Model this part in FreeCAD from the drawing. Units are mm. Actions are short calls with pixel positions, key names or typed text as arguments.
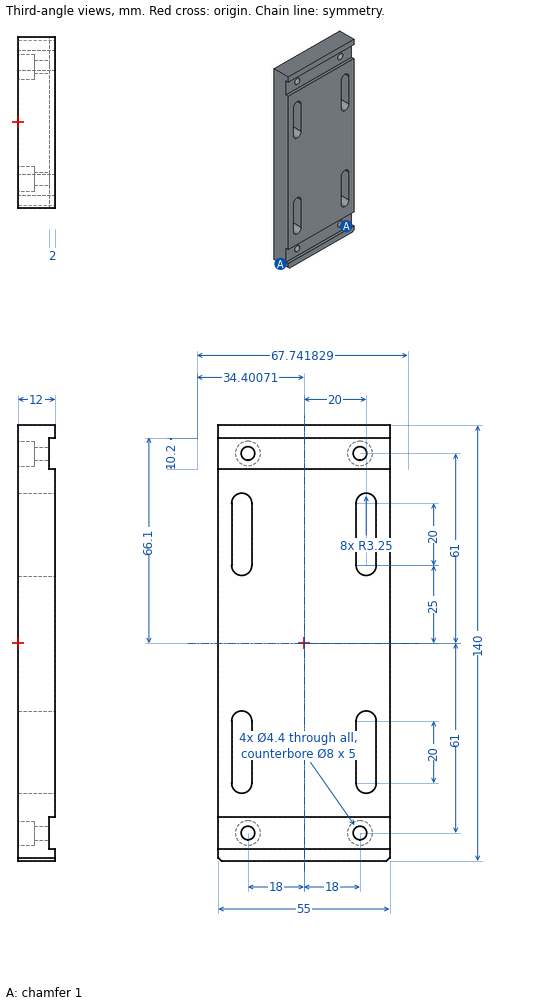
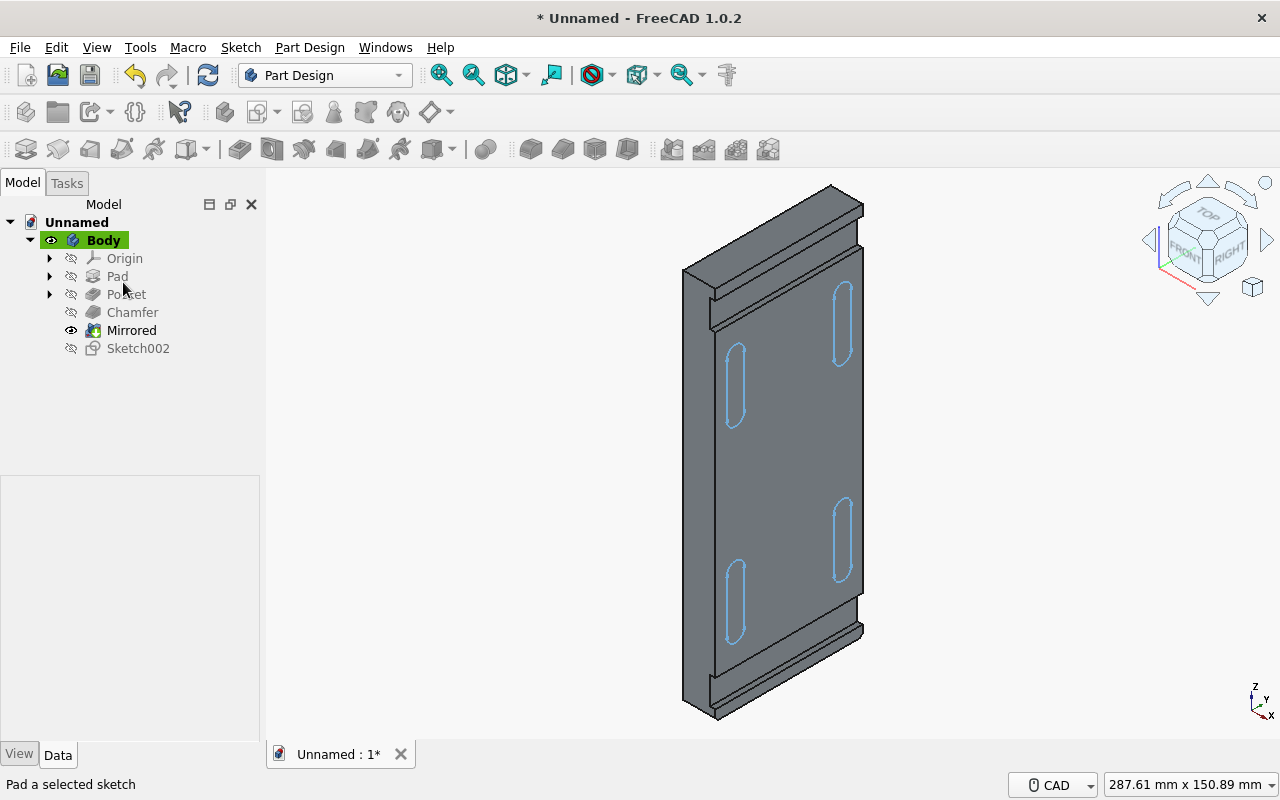
click(240, 150)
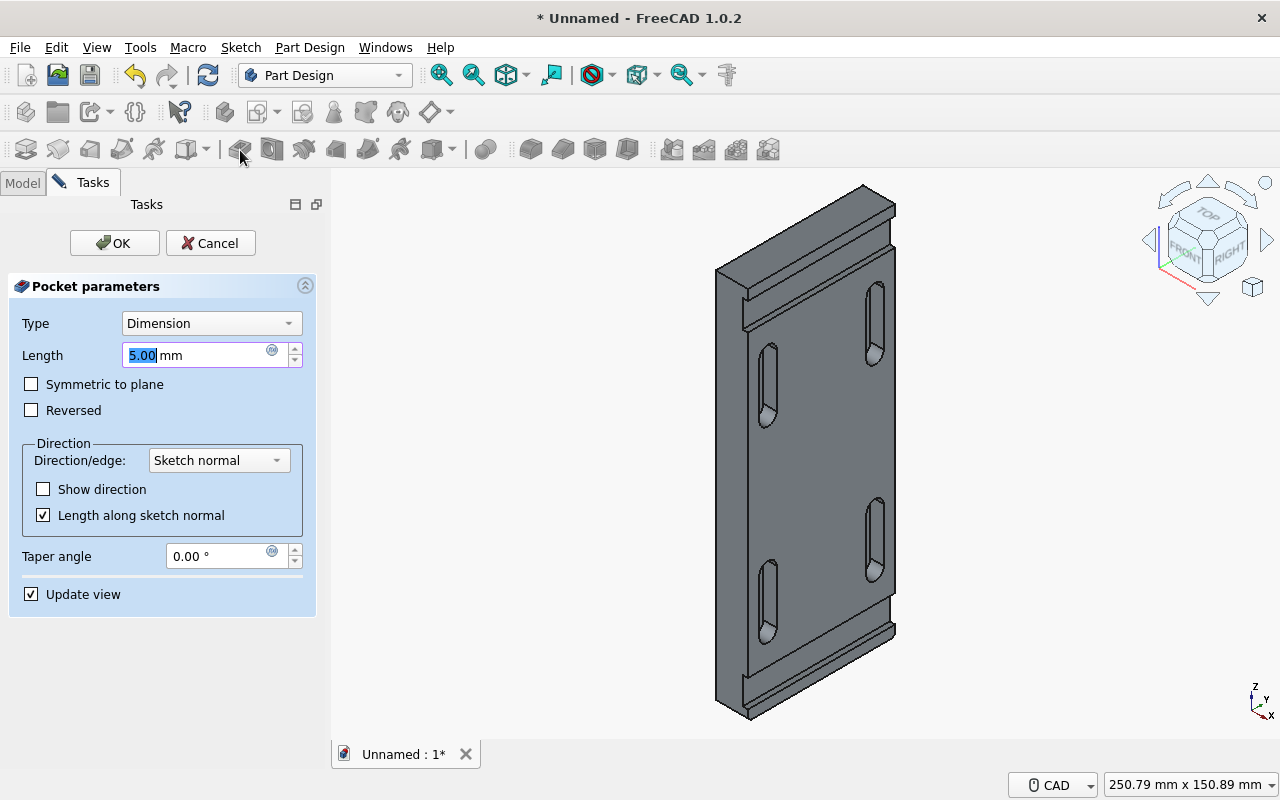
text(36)
key(Tab)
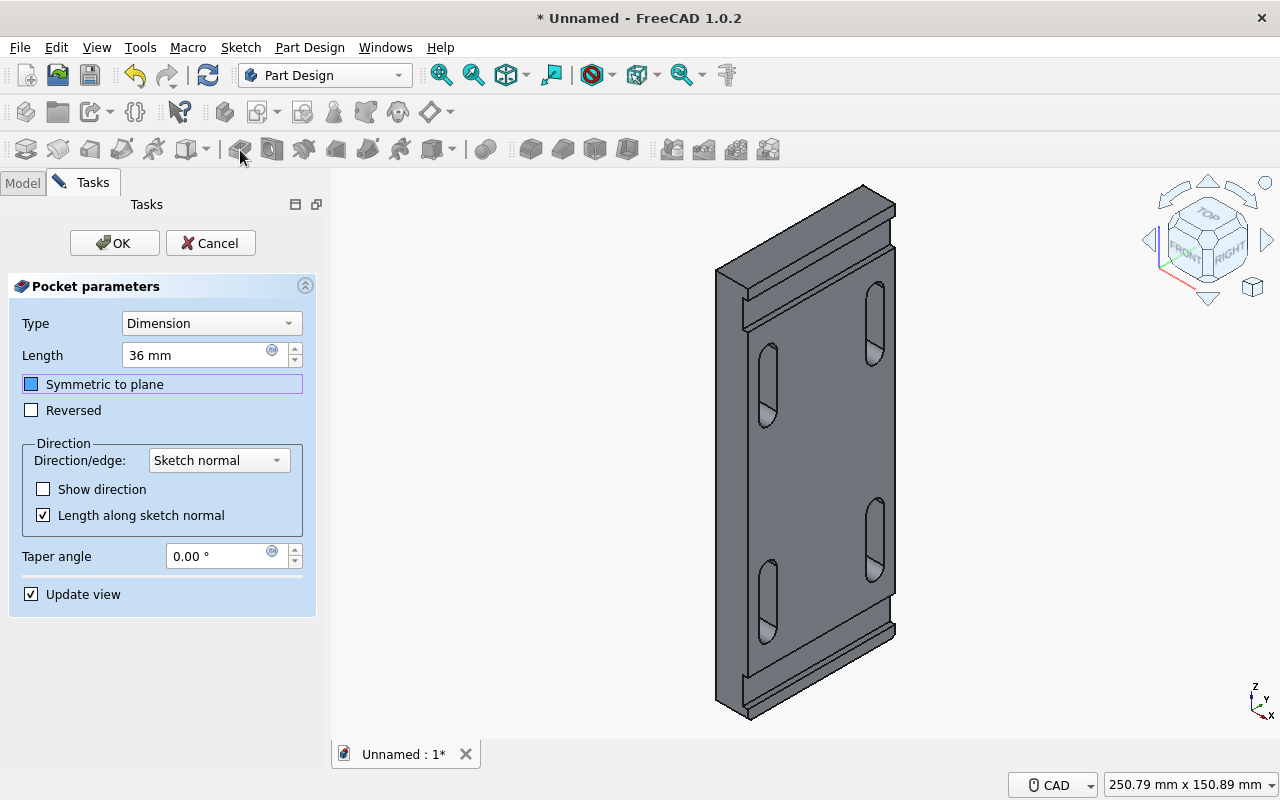
click(115, 243)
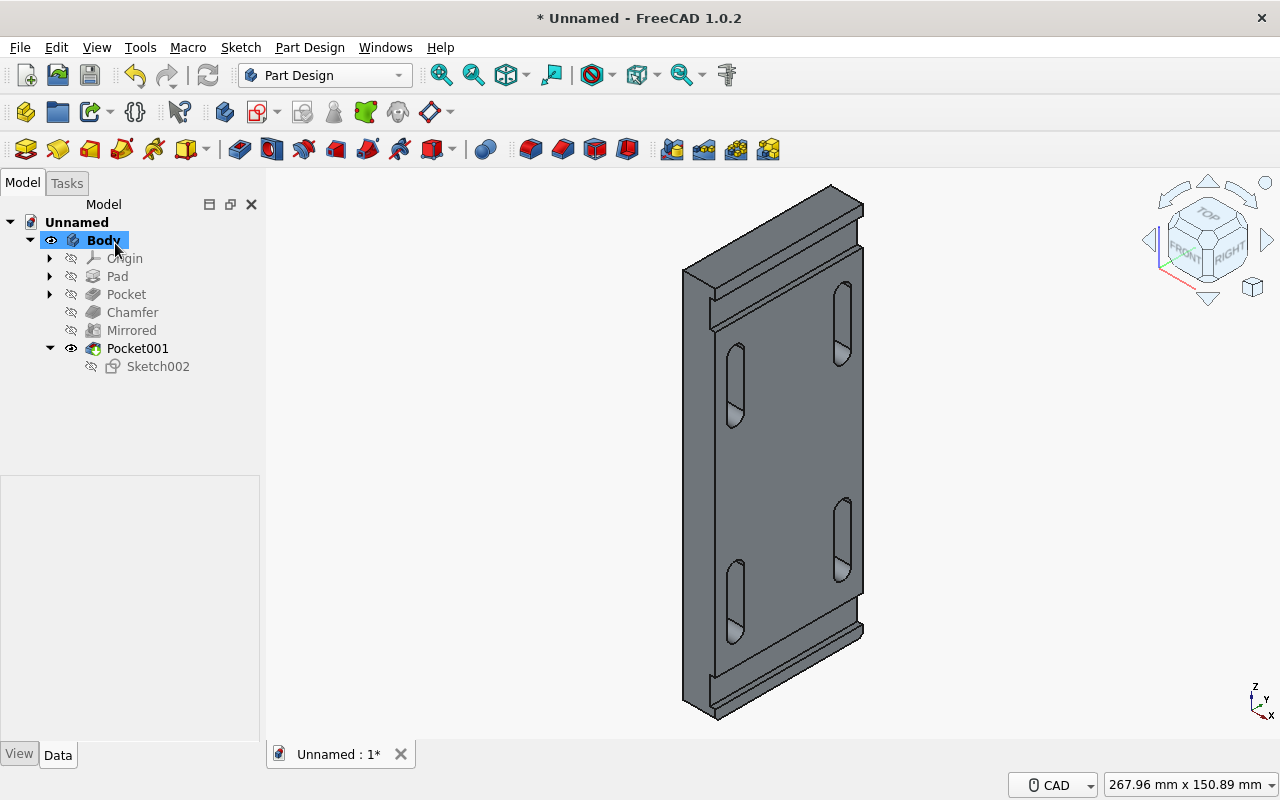
click(258, 112)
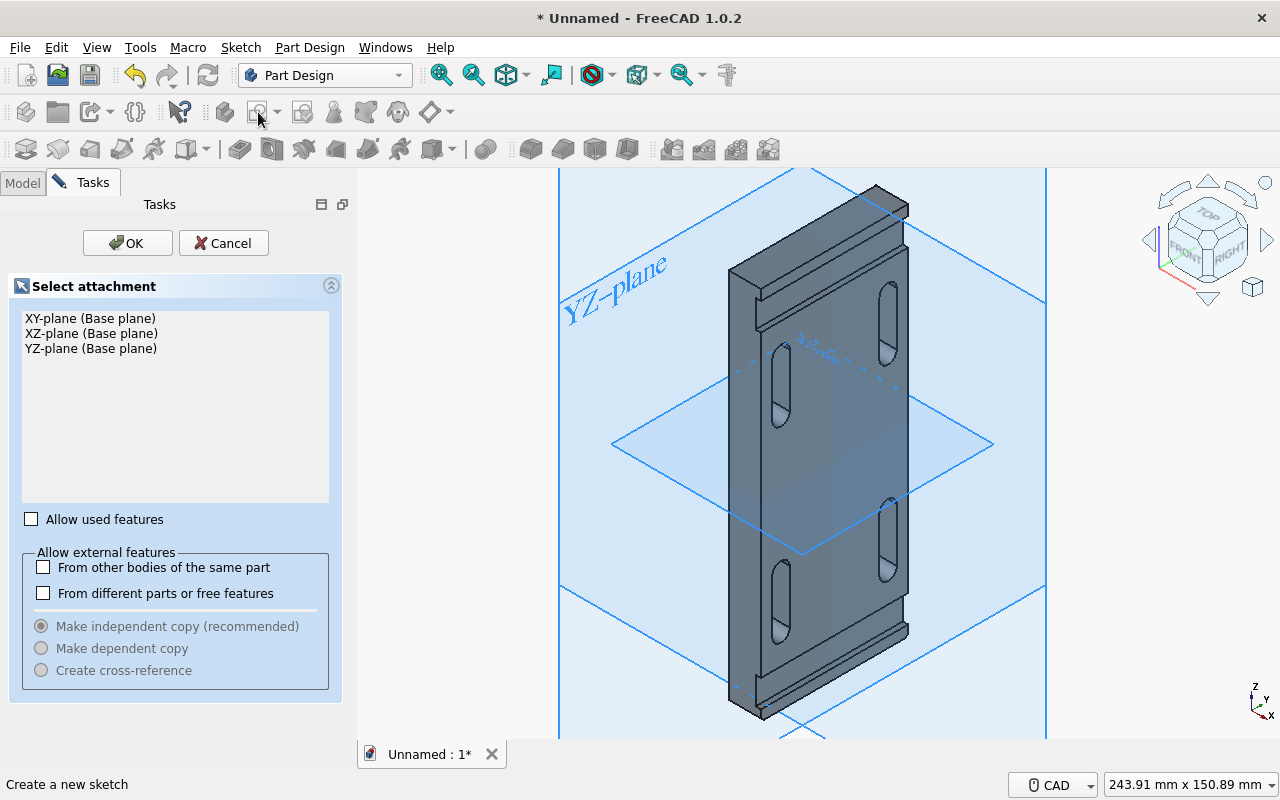
click(82, 348)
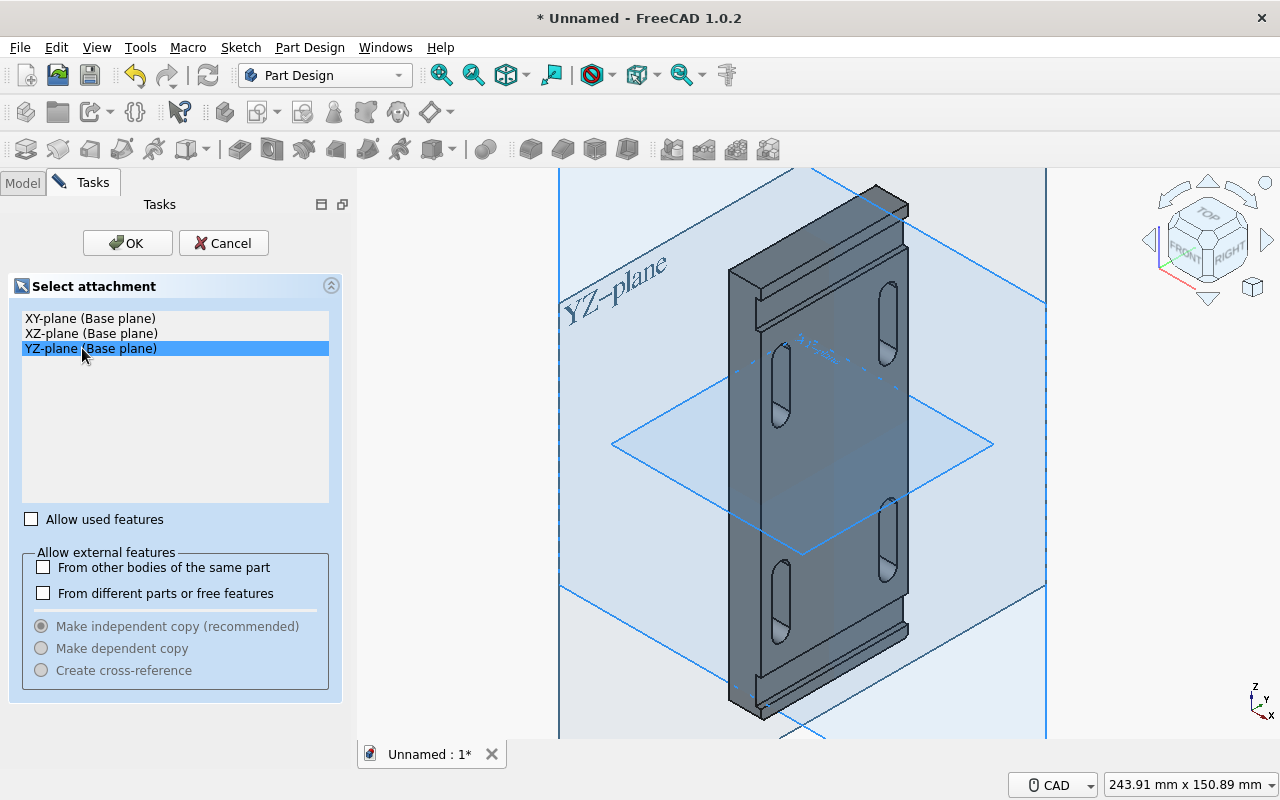
click(128, 243)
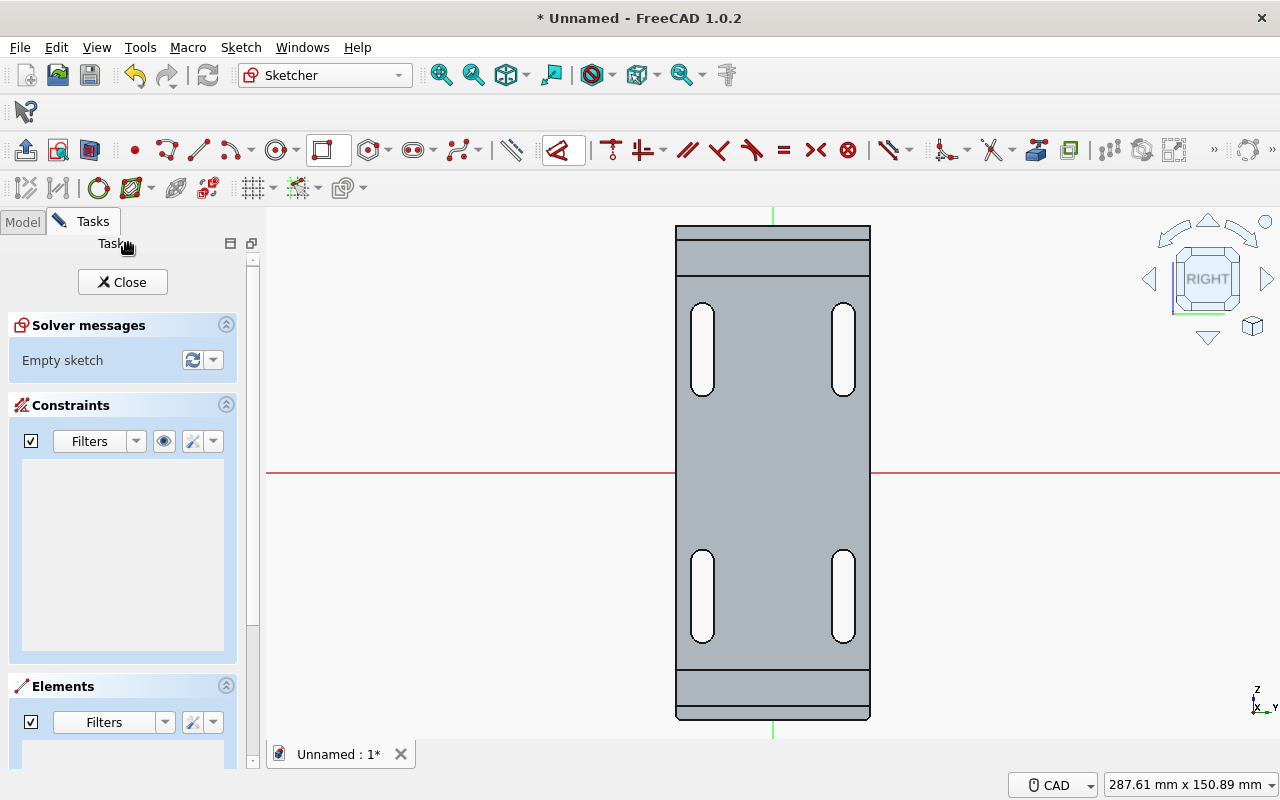
click(90, 150)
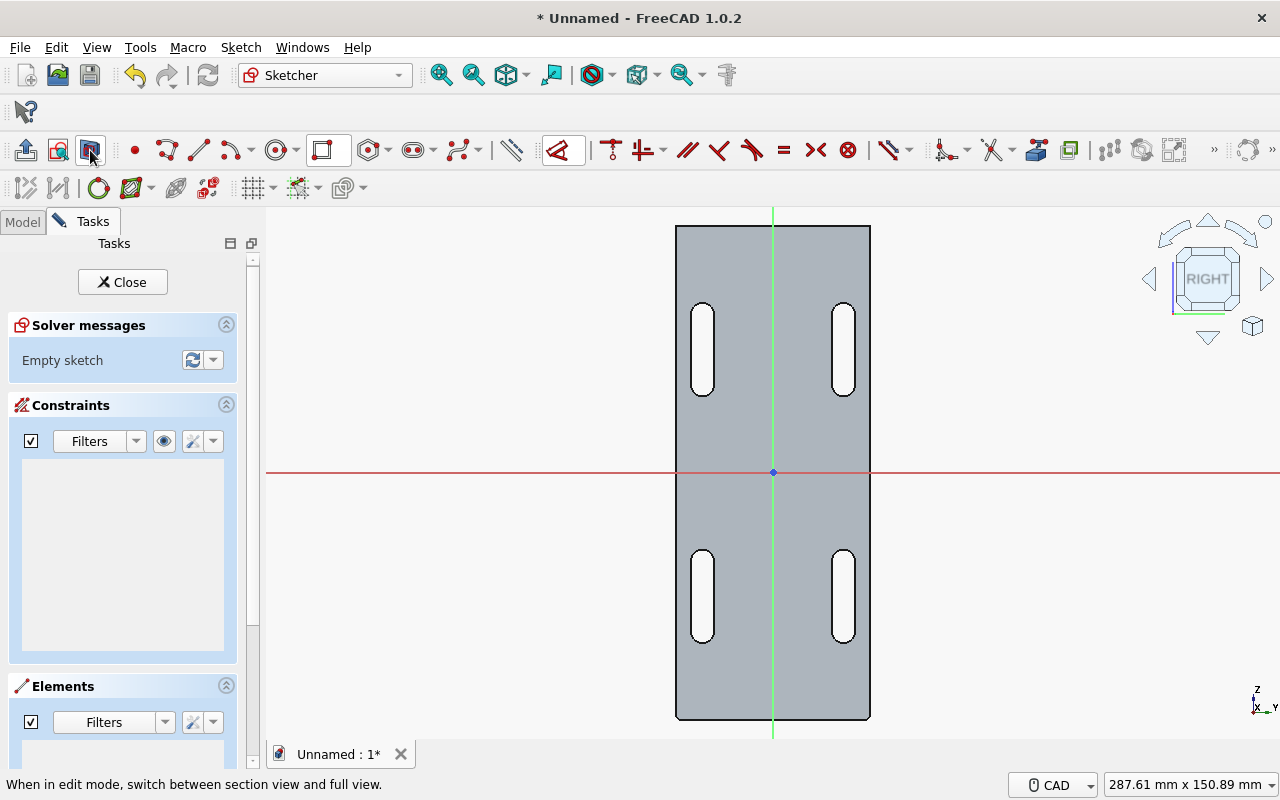
scroll(395, 473, down, 1)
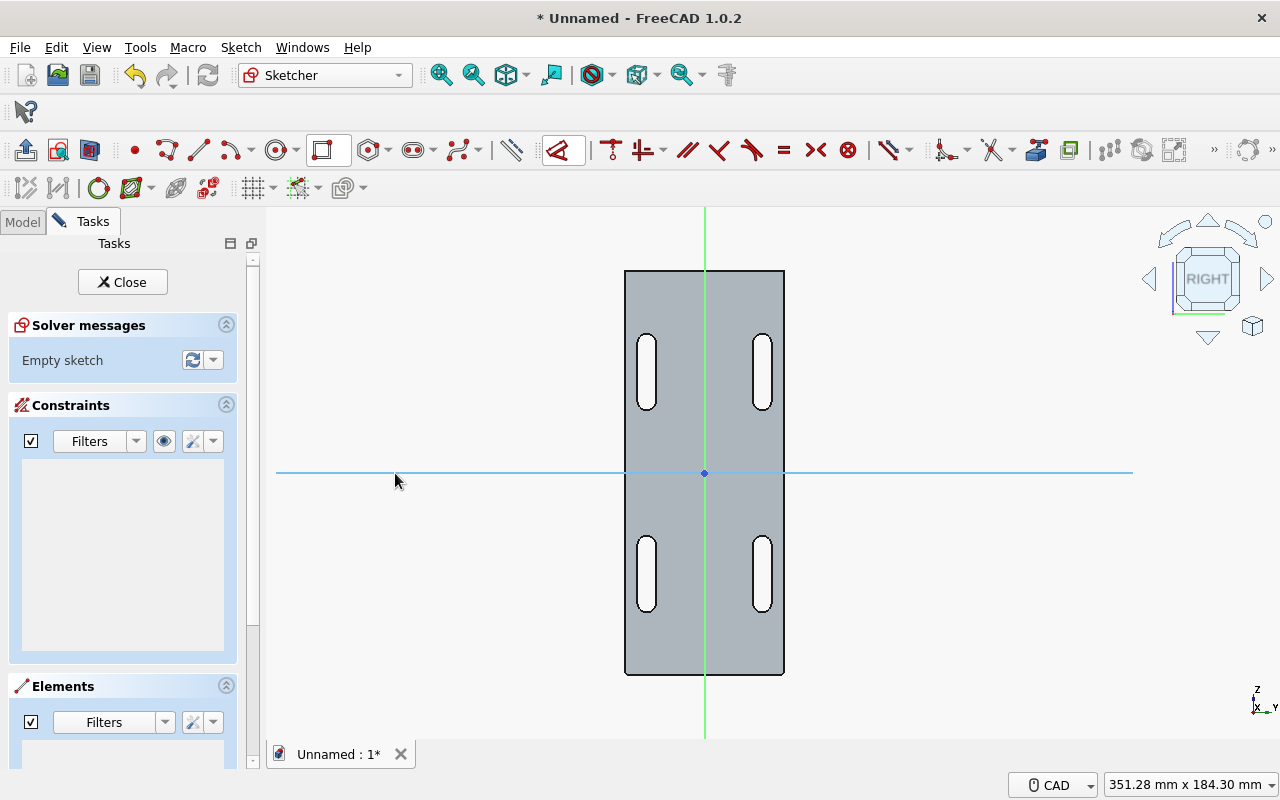
click(276, 150)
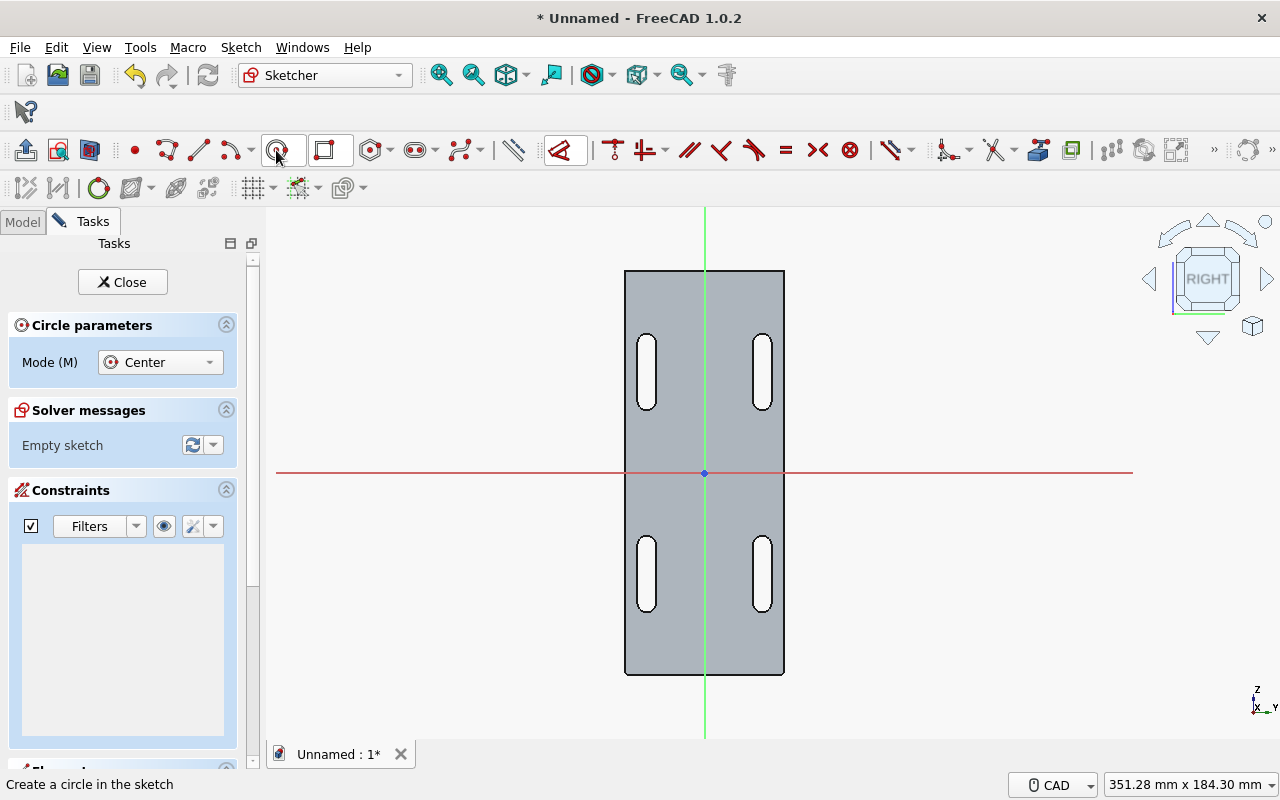
scroll(756, 649, up, 7)